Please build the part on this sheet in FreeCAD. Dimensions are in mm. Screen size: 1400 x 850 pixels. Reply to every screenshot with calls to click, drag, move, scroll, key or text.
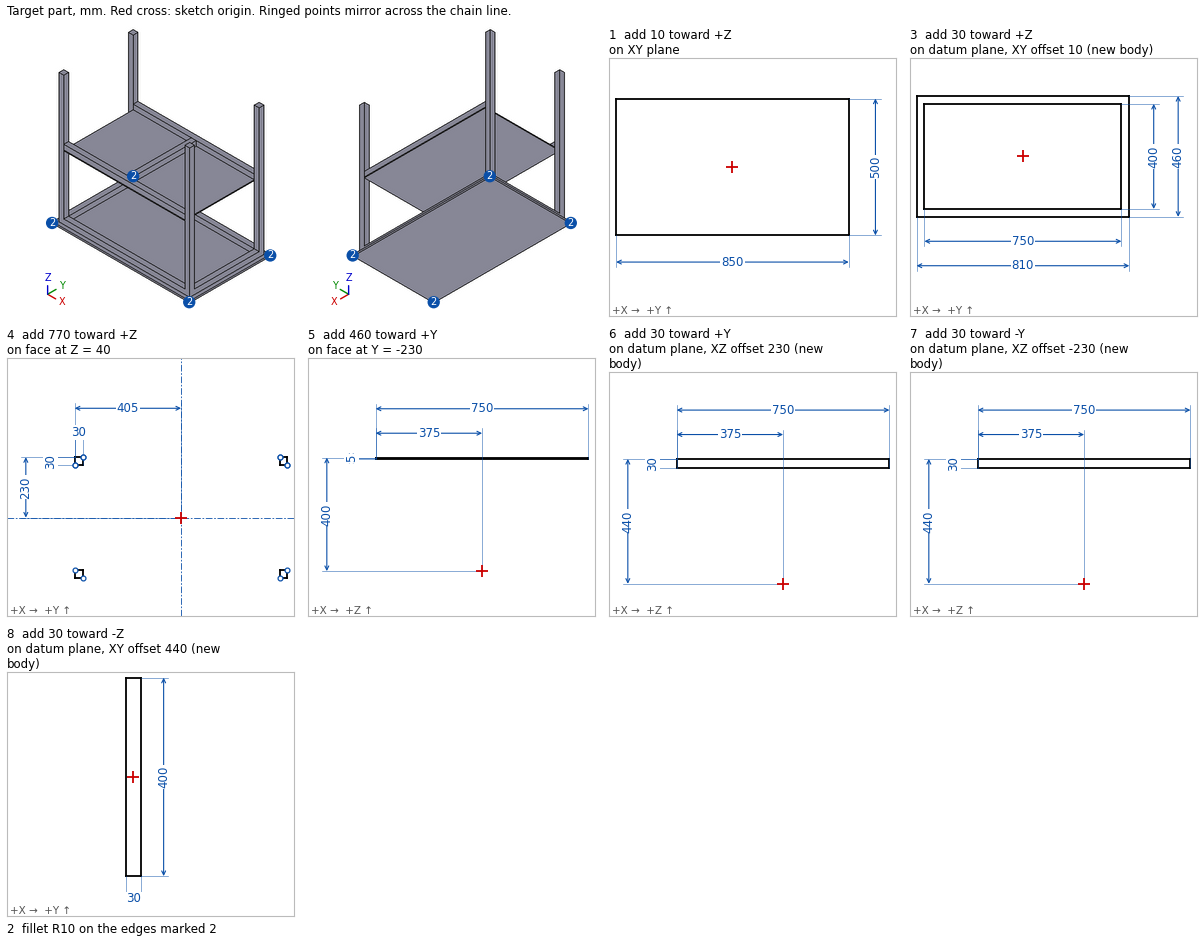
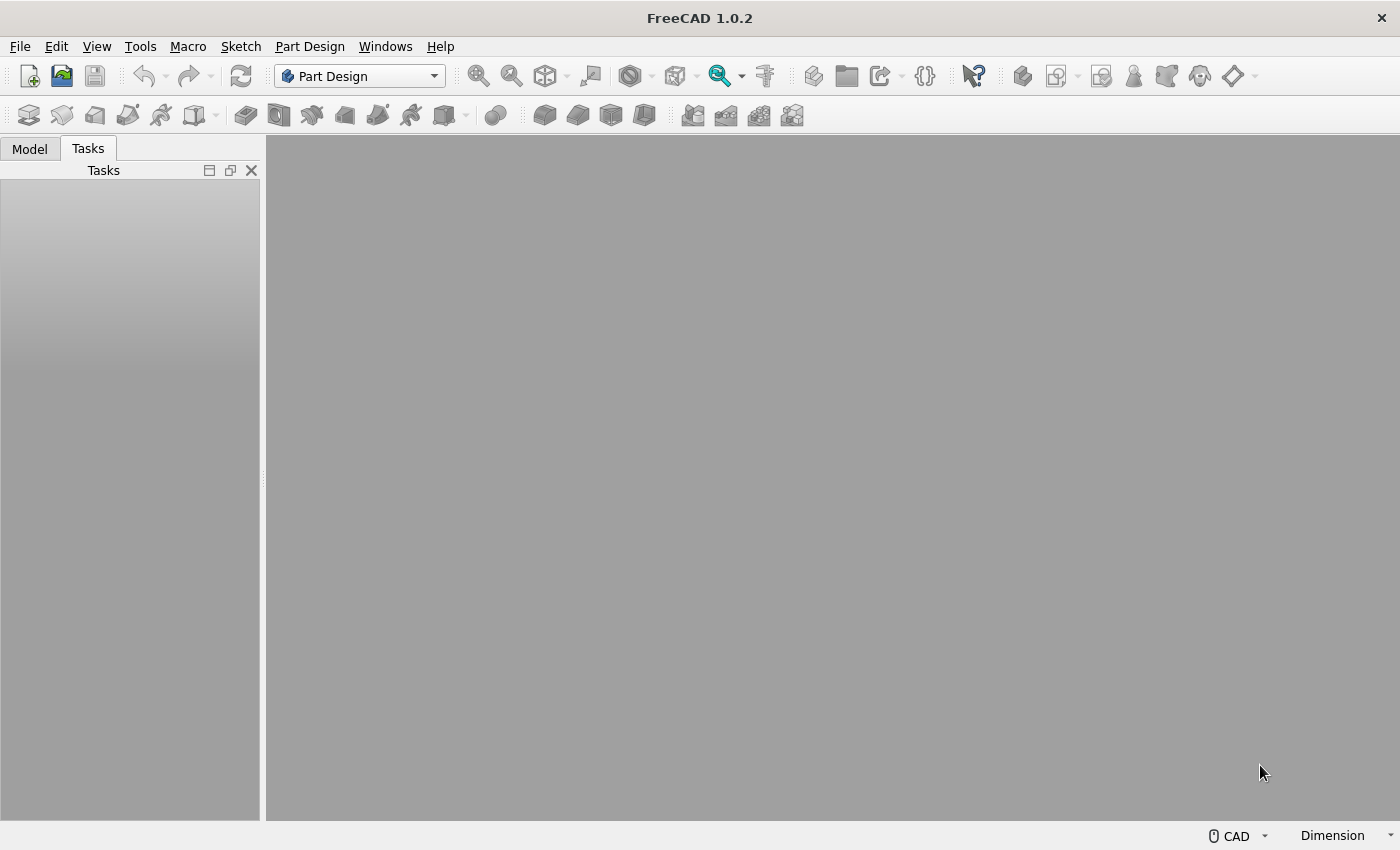
key(ctrl+n)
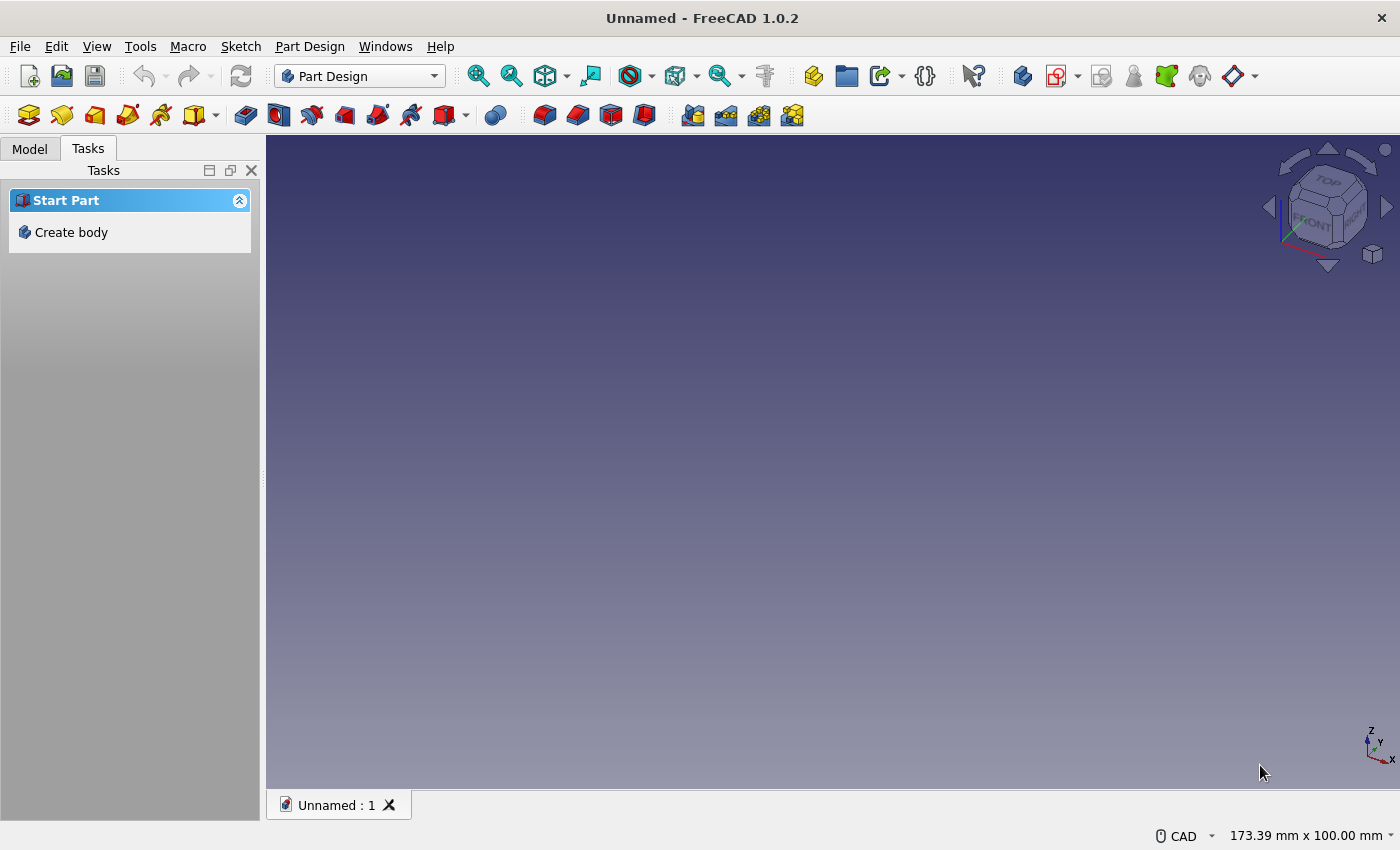
click(1056, 76)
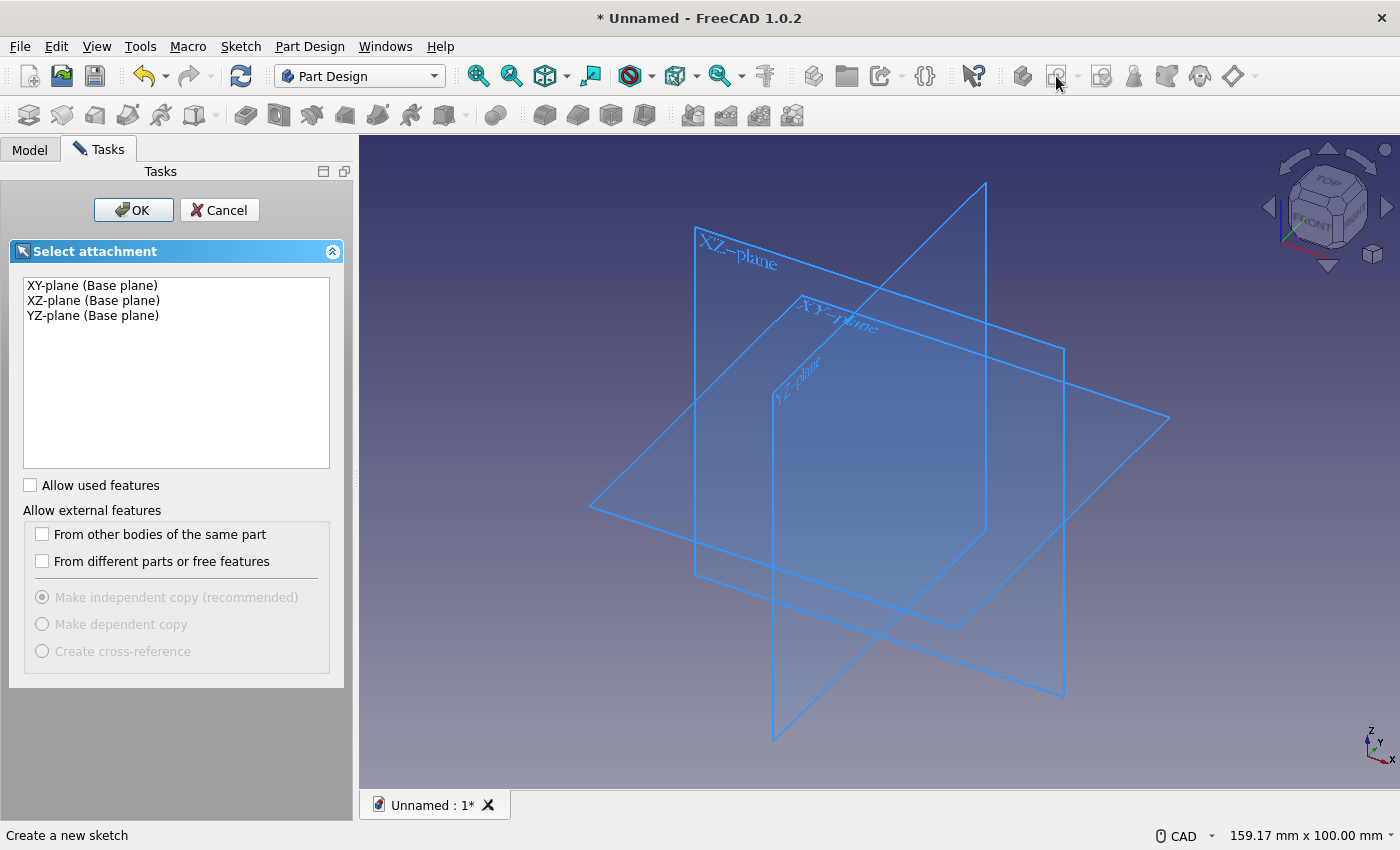
click(84, 286)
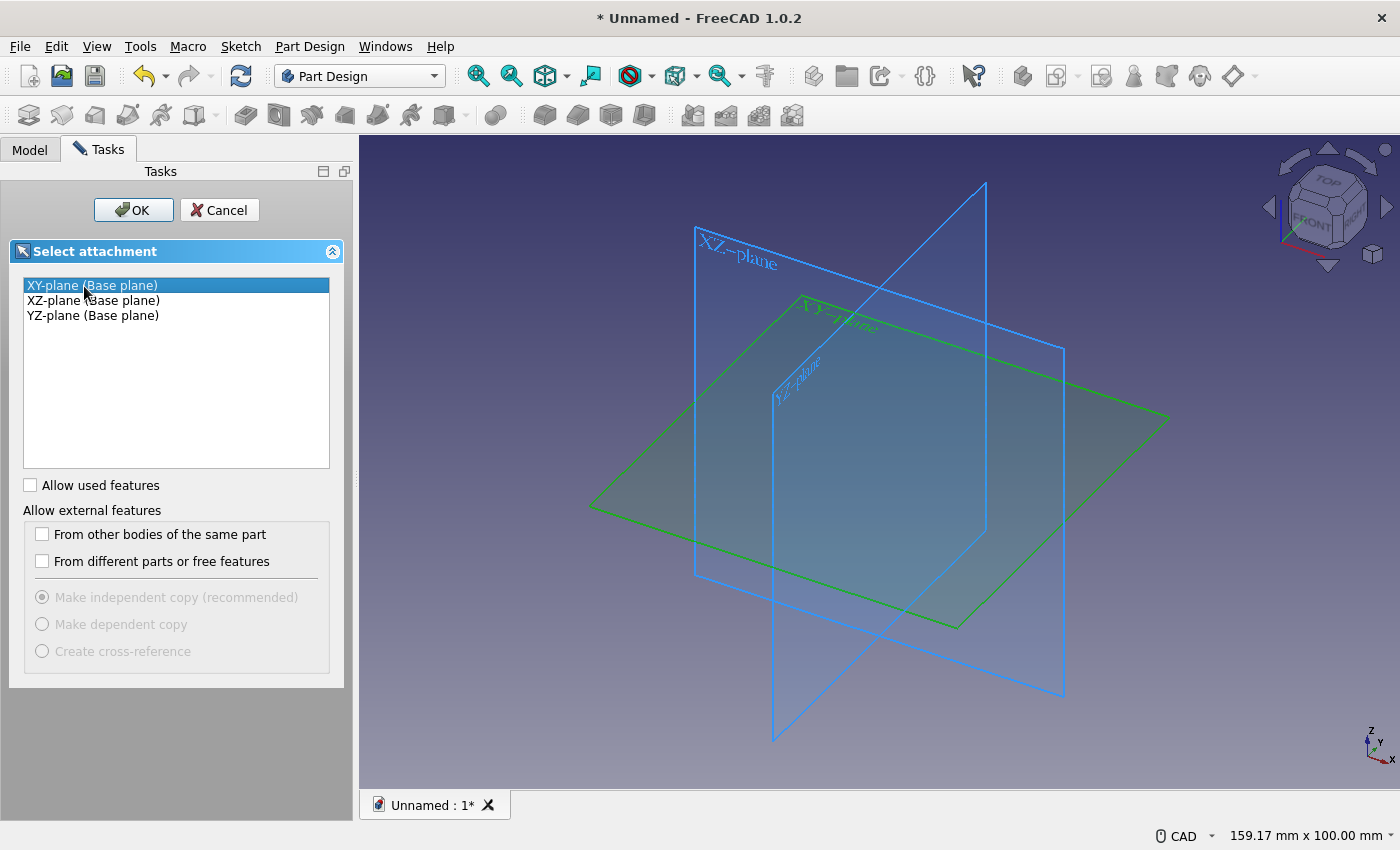
click(134, 210)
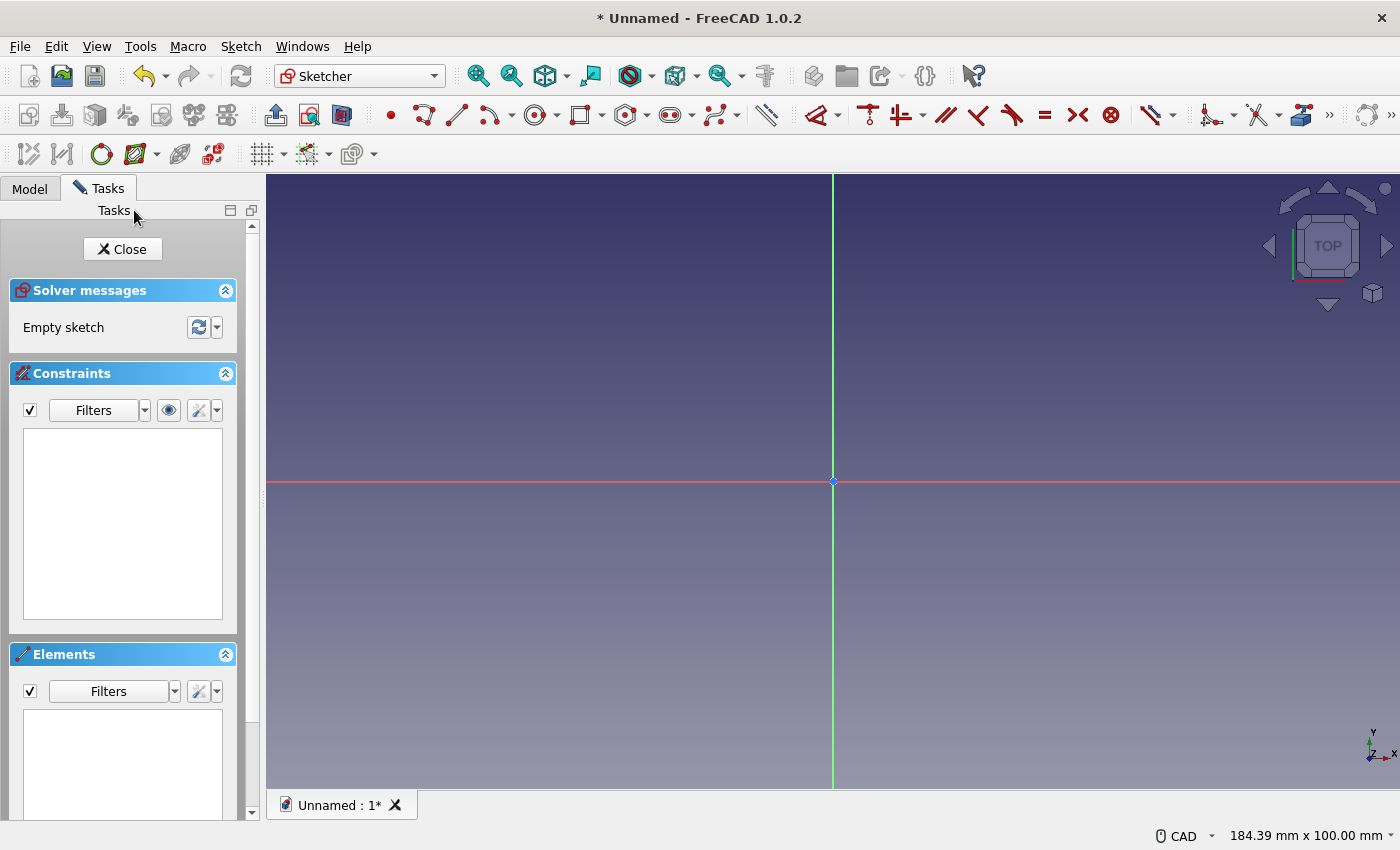
scroll(754, 482, down, 10)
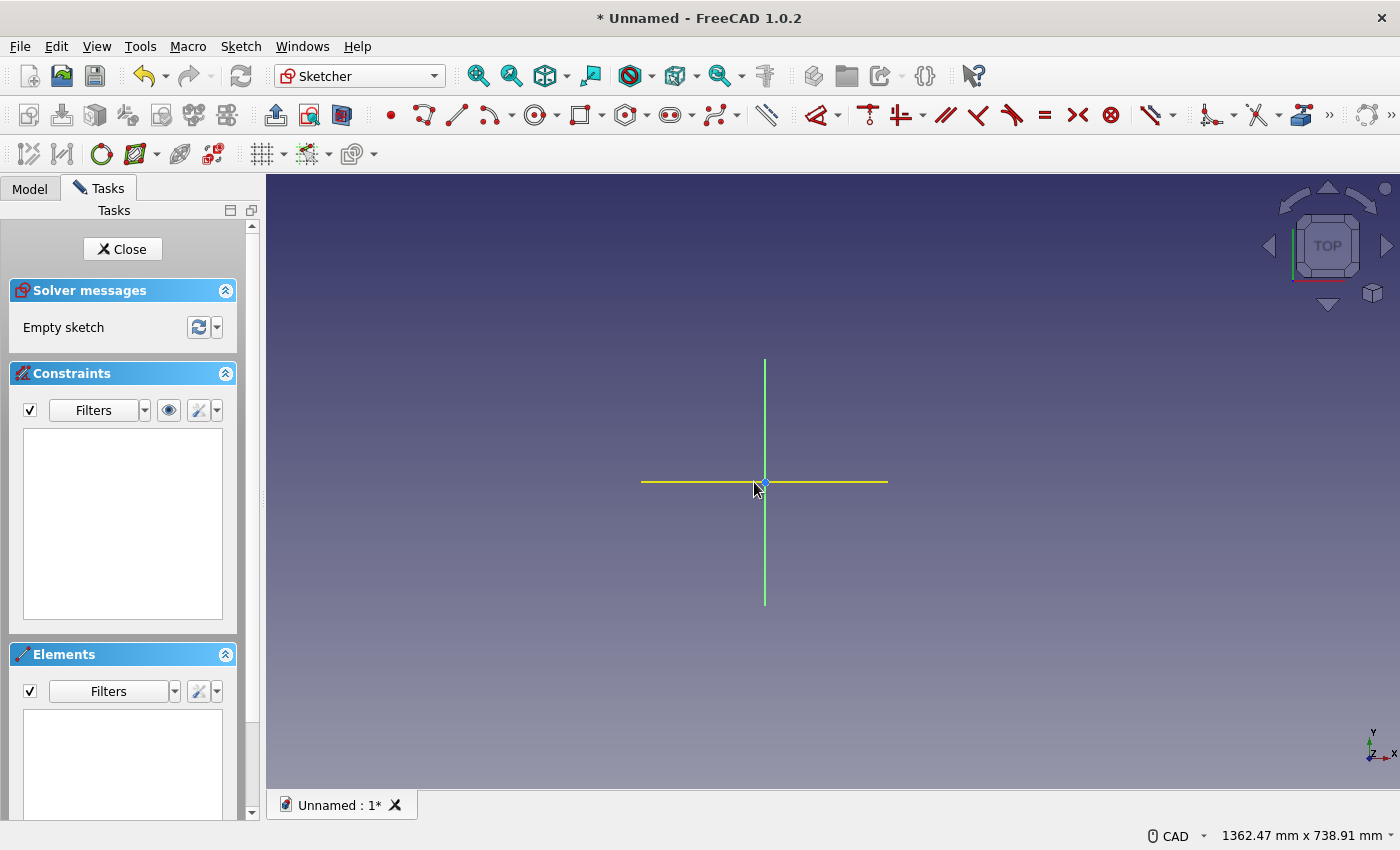
click(602, 116)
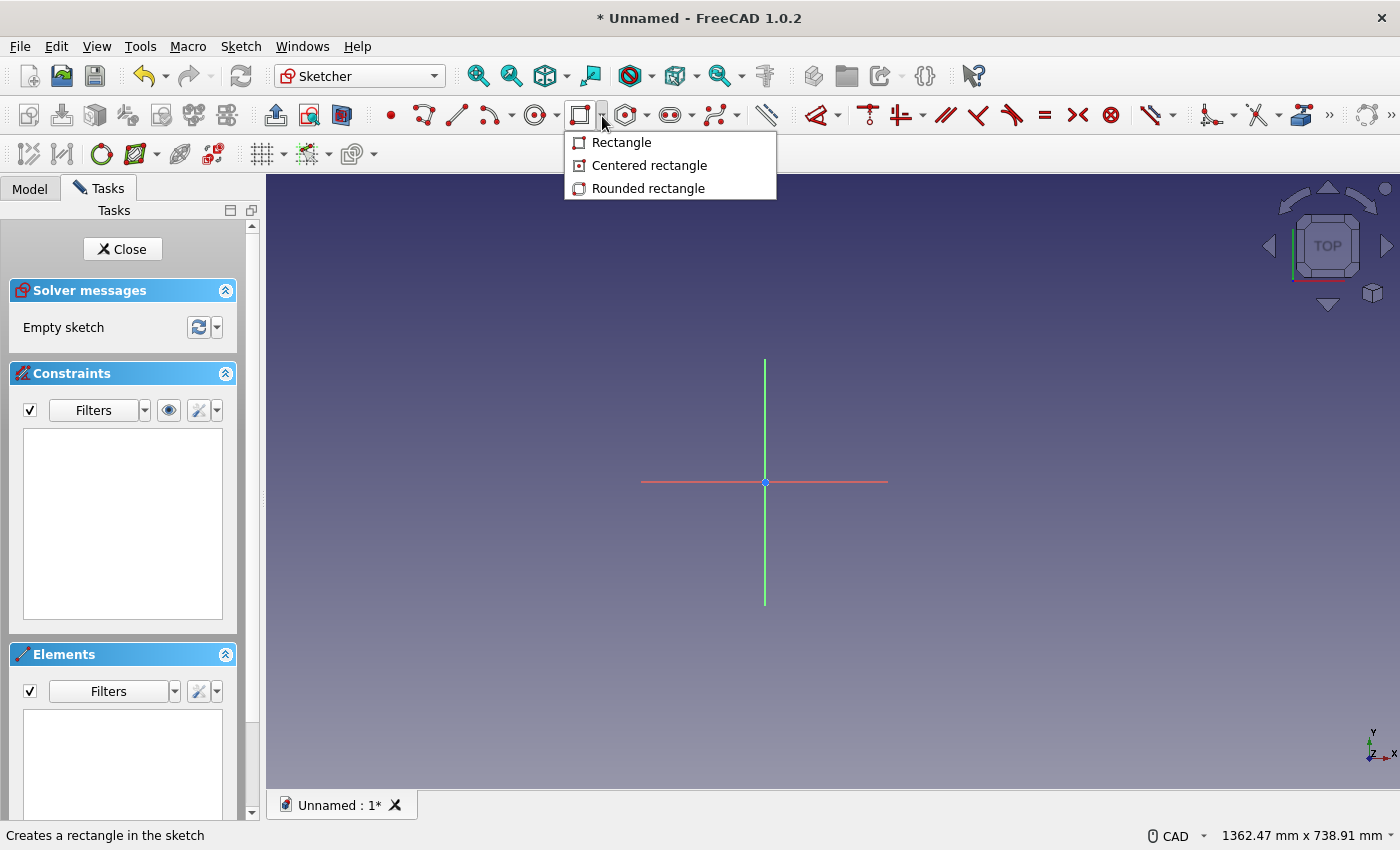
click(670, 166)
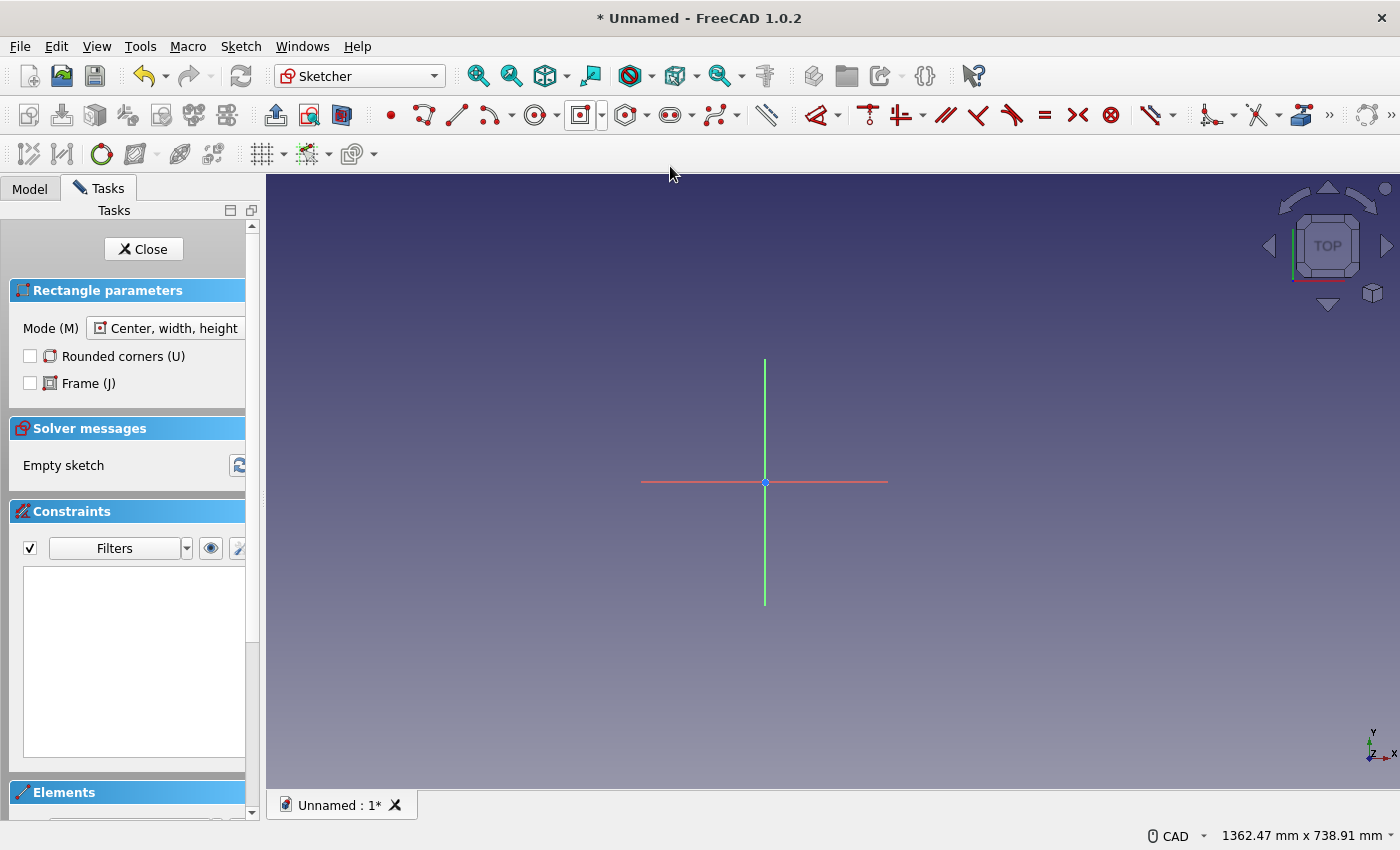
click(765, 482)
click(1119, 274)
key(Escape)